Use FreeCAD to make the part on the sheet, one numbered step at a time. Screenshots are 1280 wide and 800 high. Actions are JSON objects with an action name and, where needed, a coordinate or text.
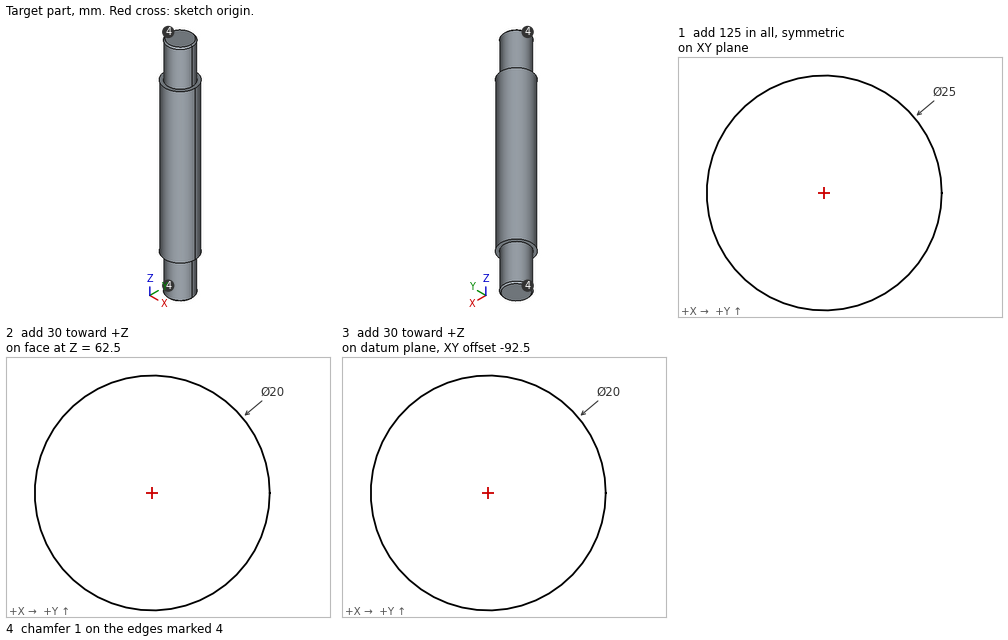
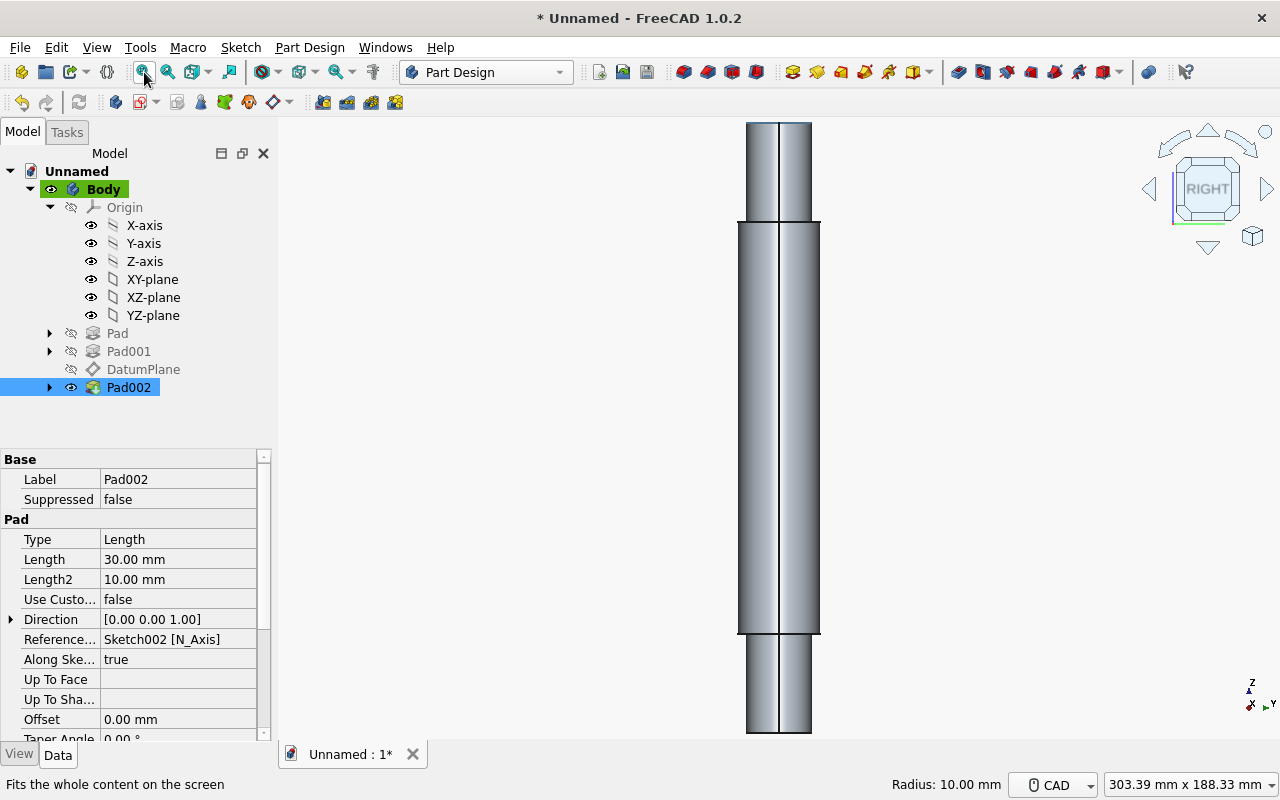
{"action": "key", "text": "5"}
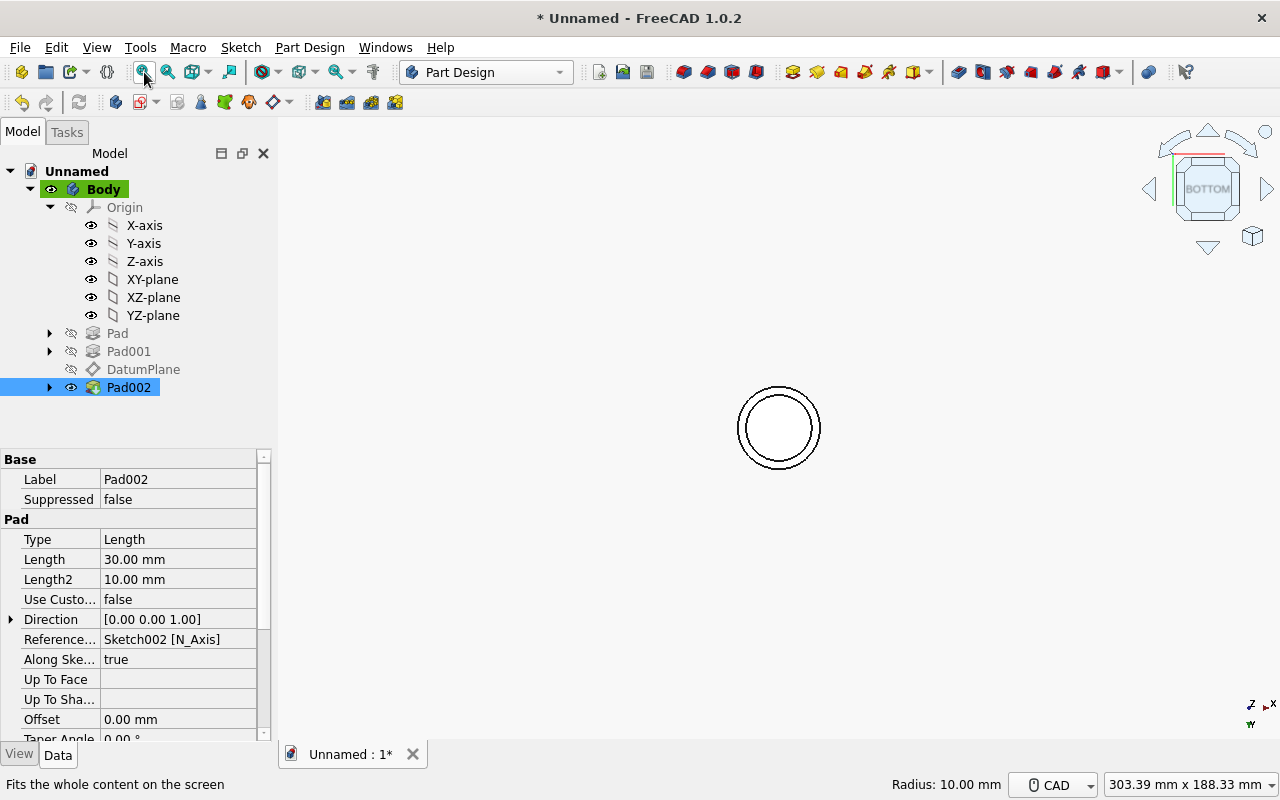
{"action": "left_click", "coordinate": [144, 72]}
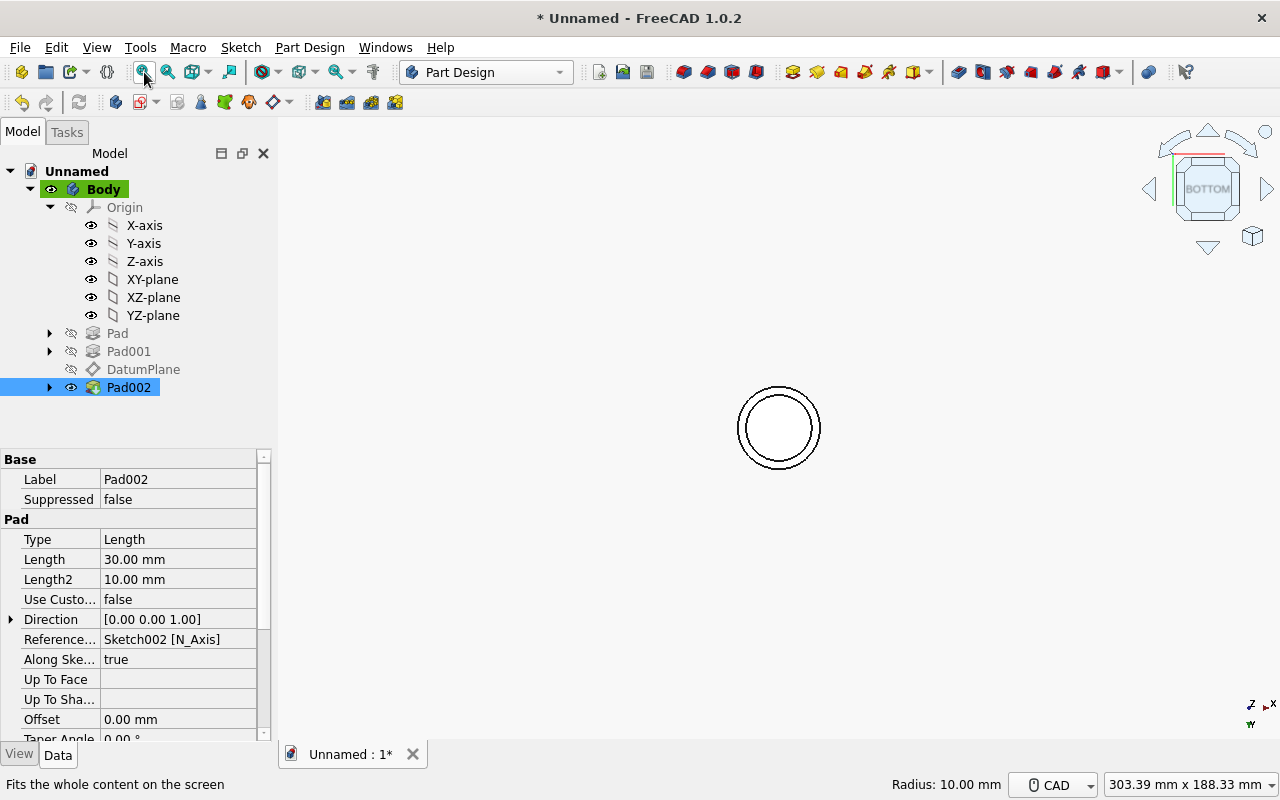
{"action": "left_click", "coordinate": [746, 427], "text": "ctrl"}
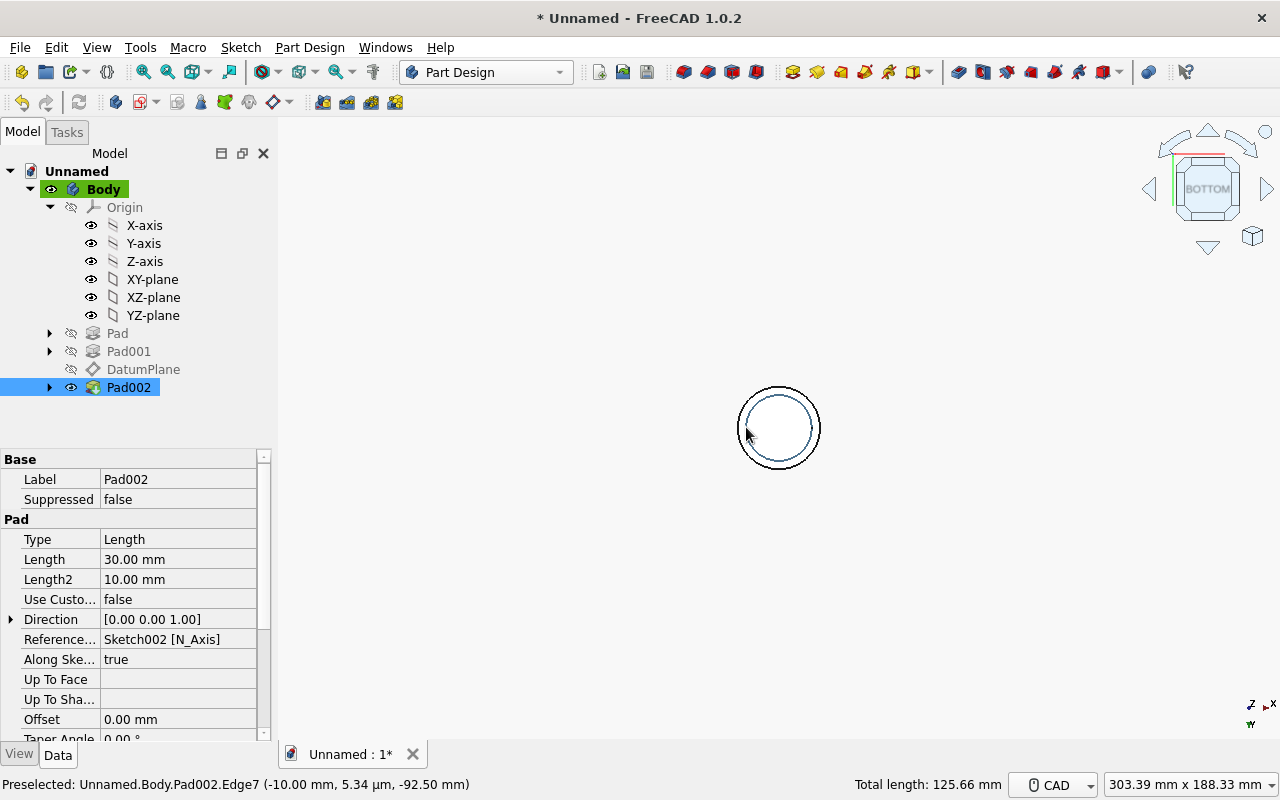
{"action": "left_click", "coordinate": [708, 72]}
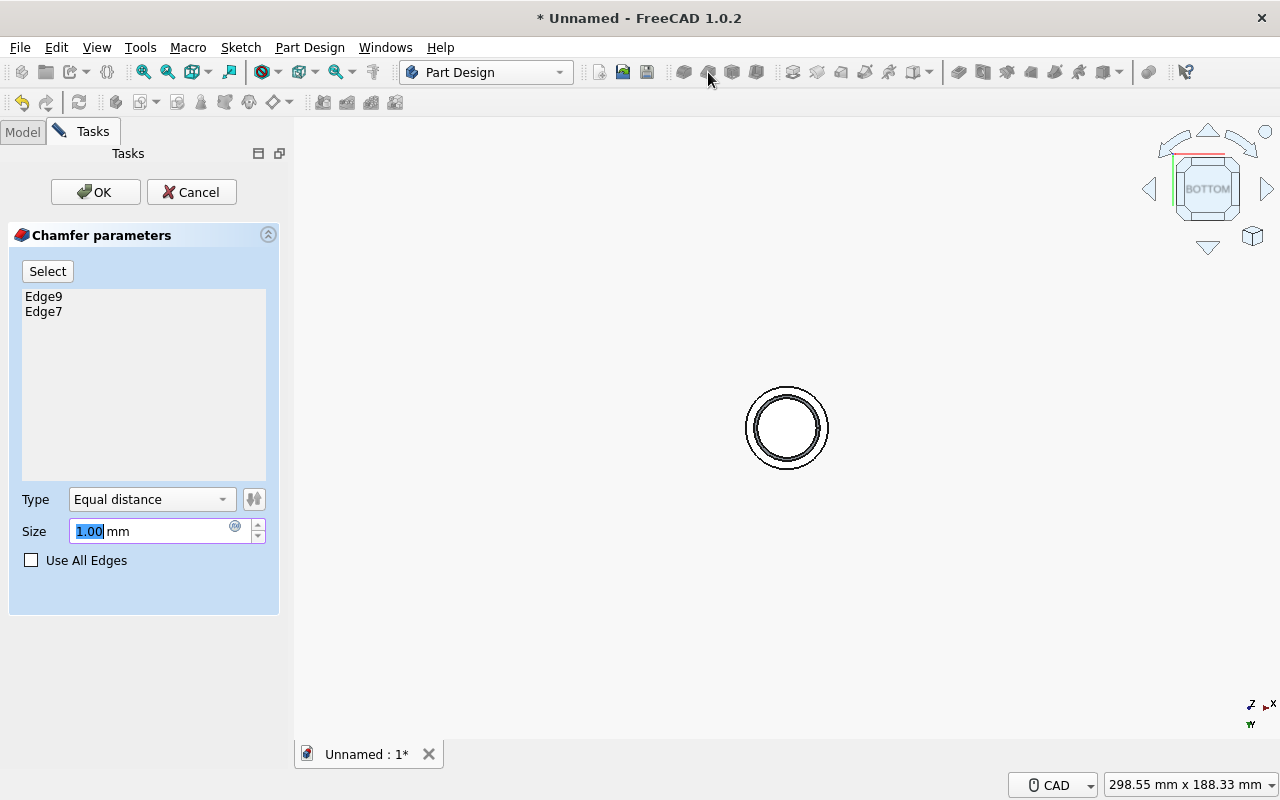
{"action": "type", "text": "1"}
{"action": "key", "text": "Tab"}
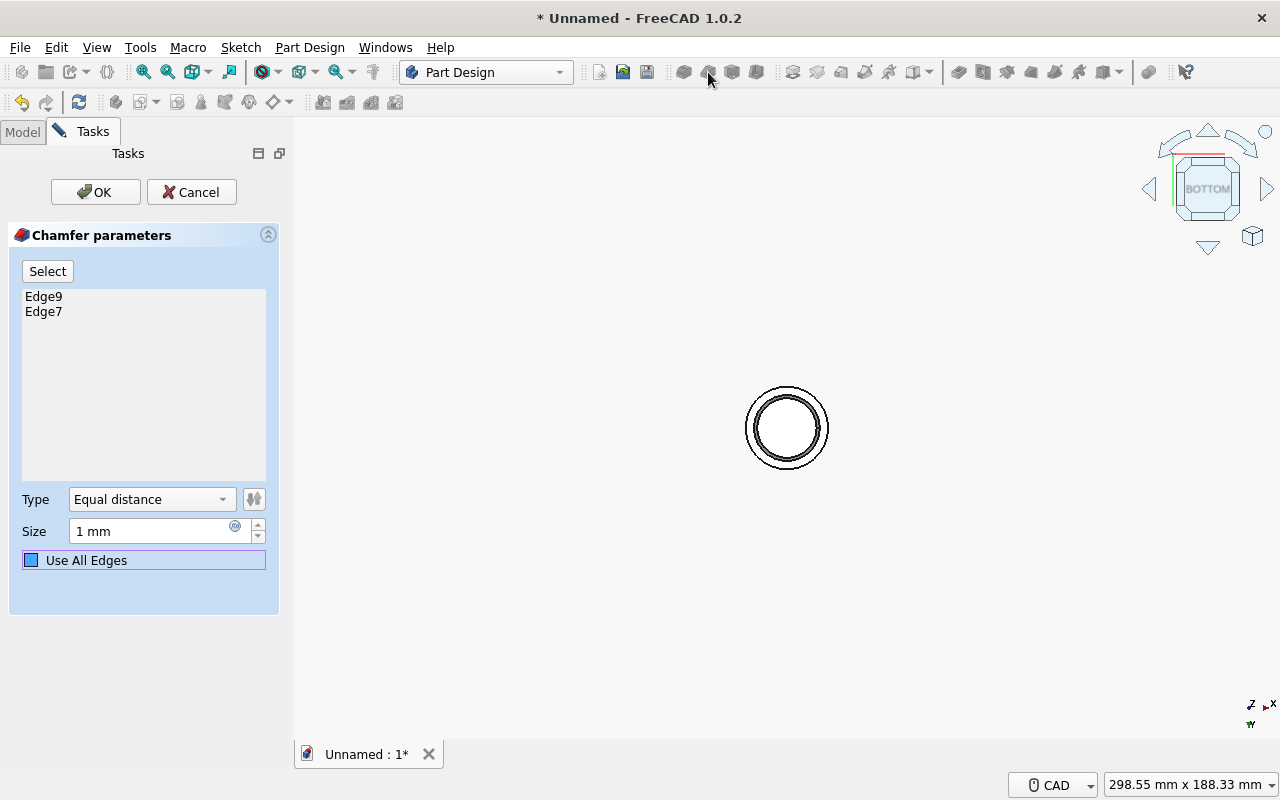
{"action": "left_click", "coordinate": [96, 192]}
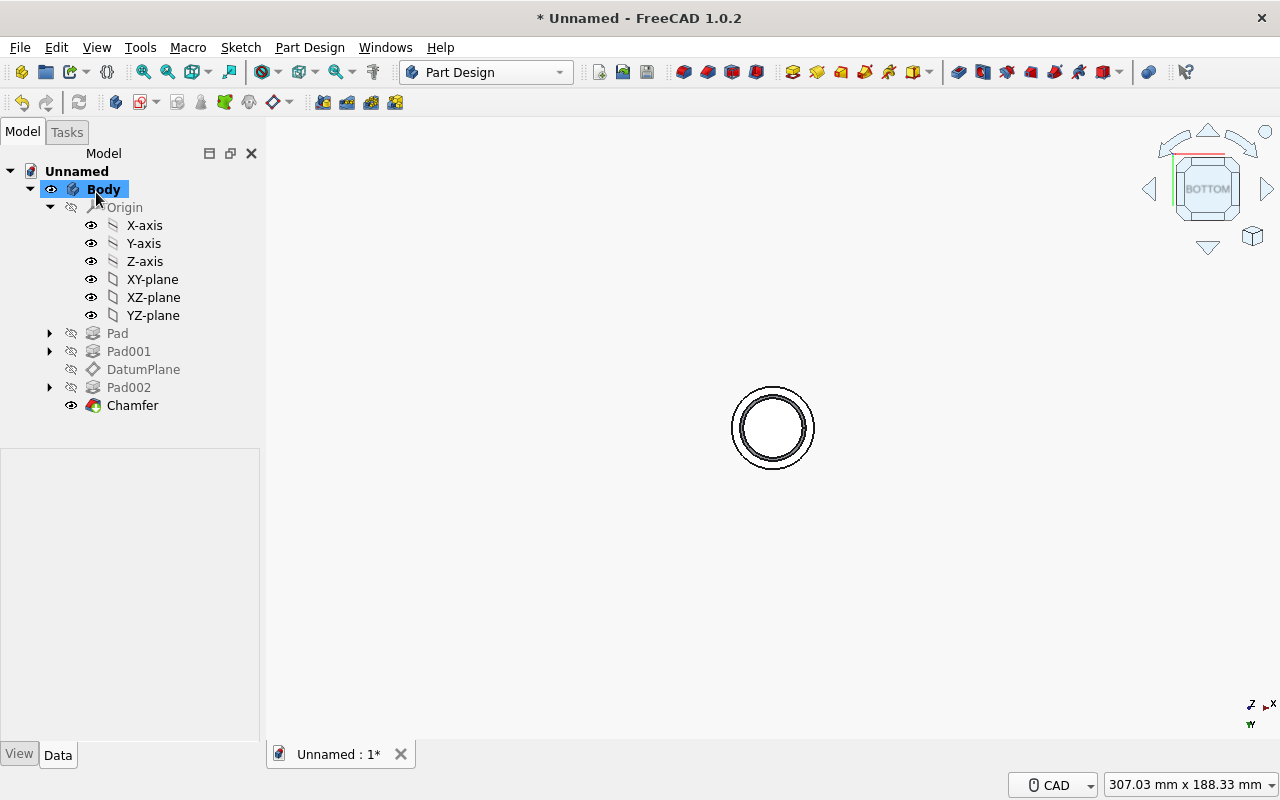
{"action": "key", "text": "0"}